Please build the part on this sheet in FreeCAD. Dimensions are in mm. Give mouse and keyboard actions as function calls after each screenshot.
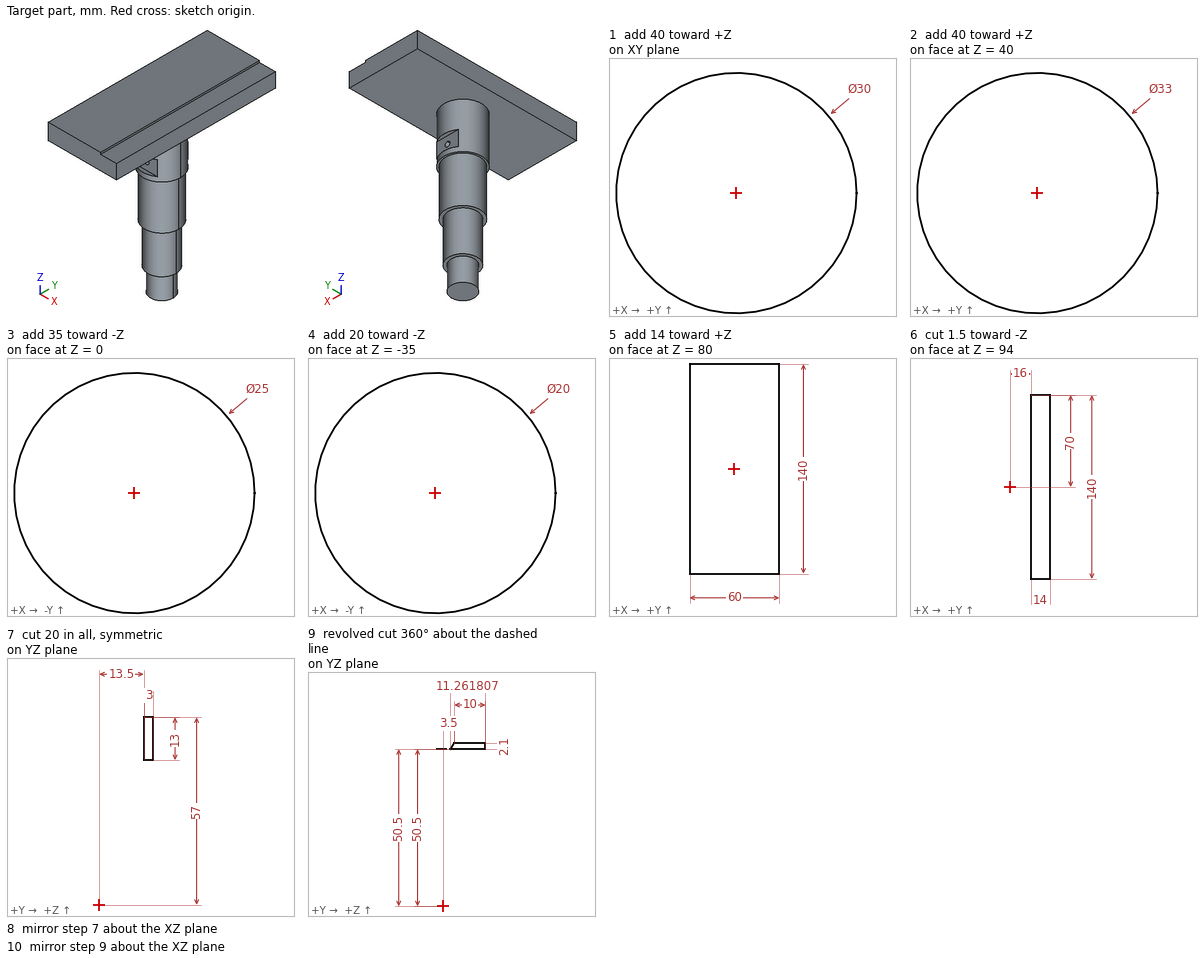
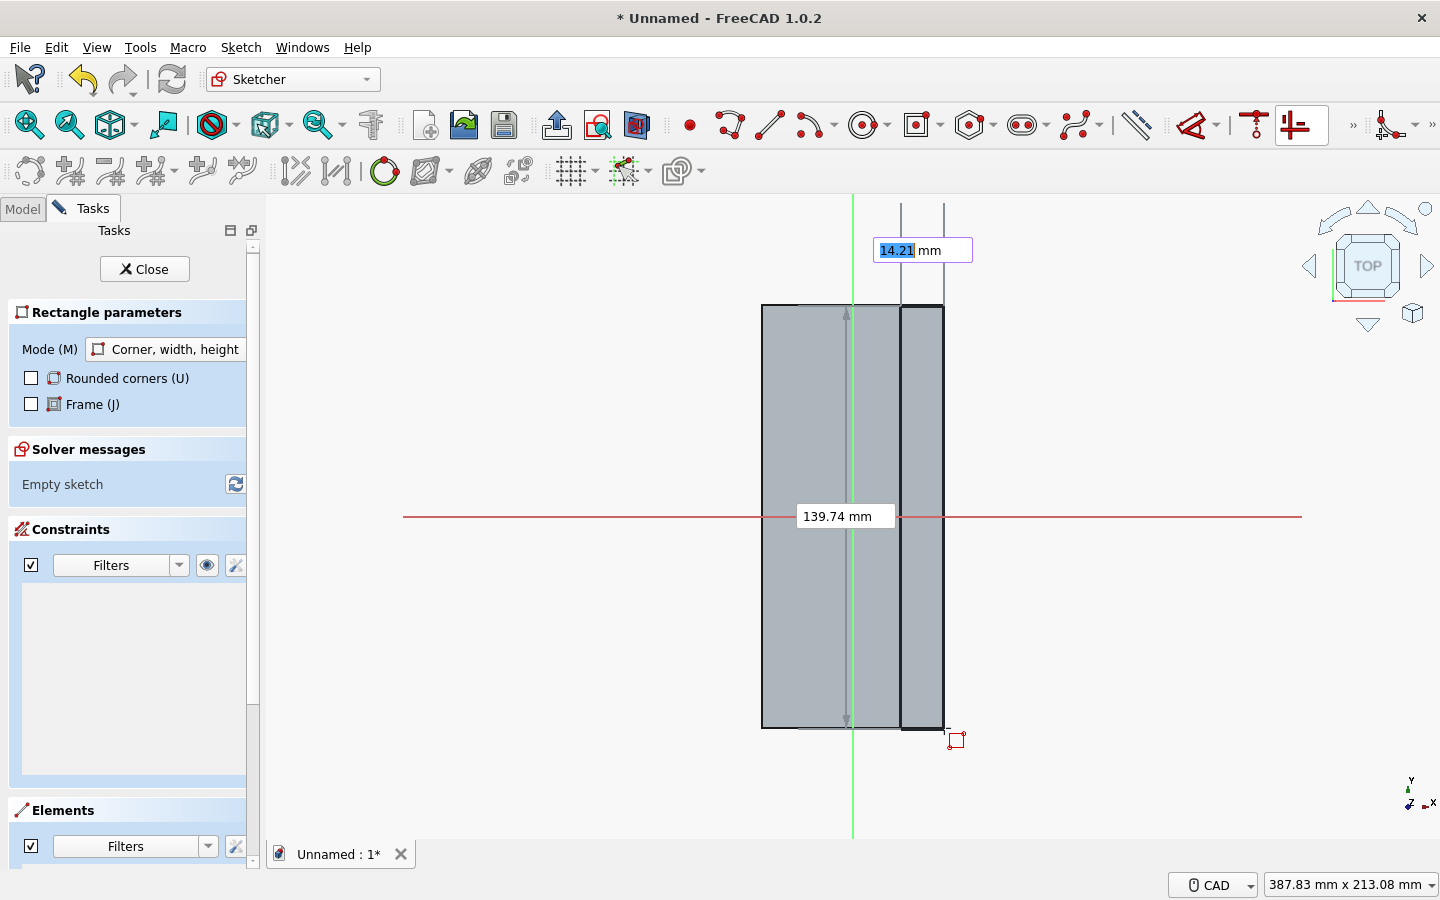
text(14)
key(Tab)
text(140)
key(Return)
key(Escape)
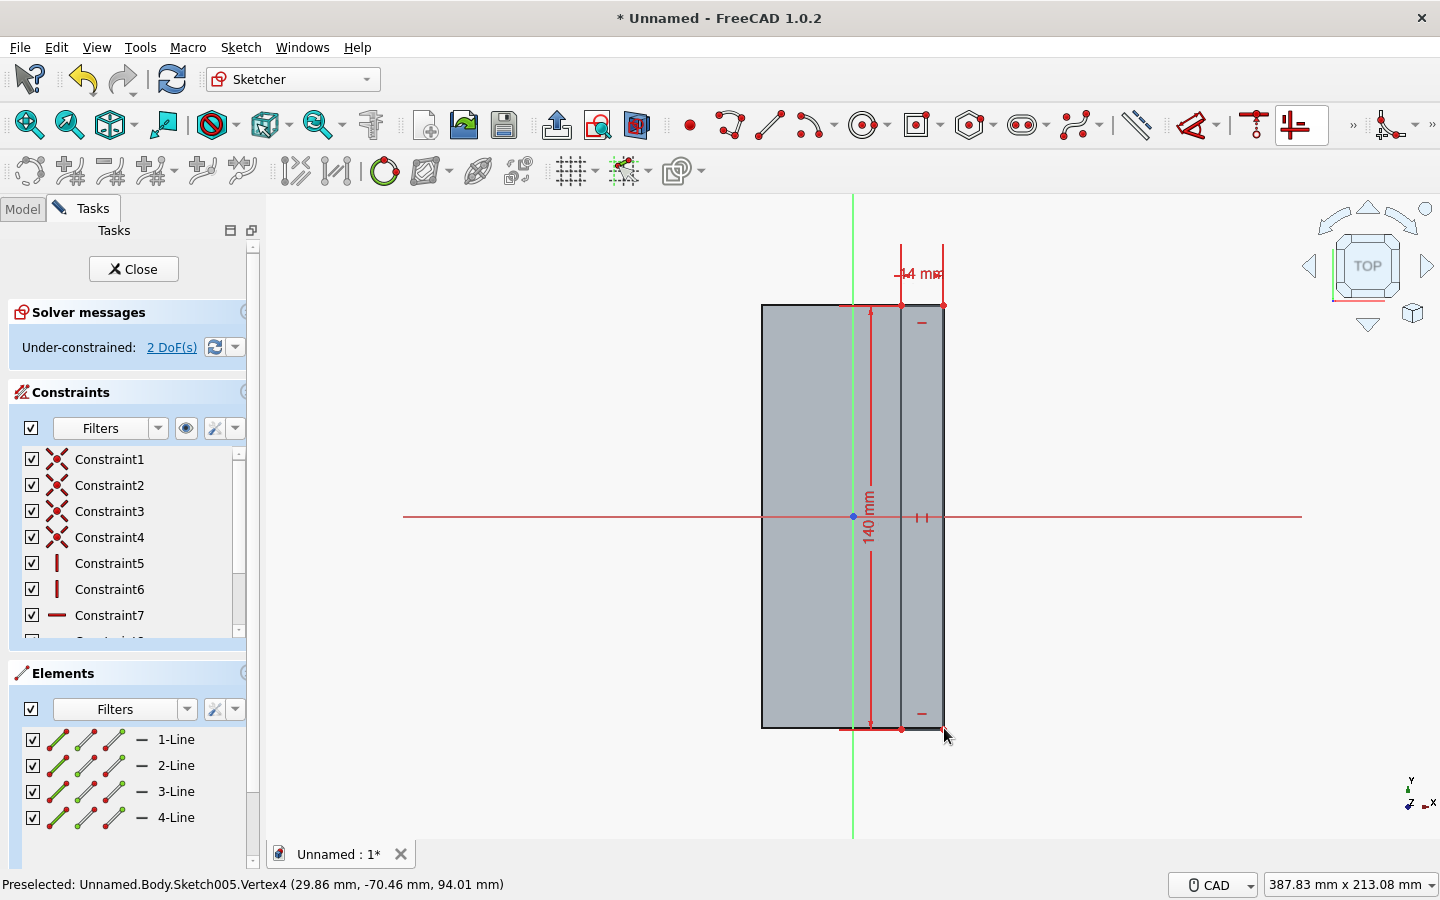
click(1192, 126)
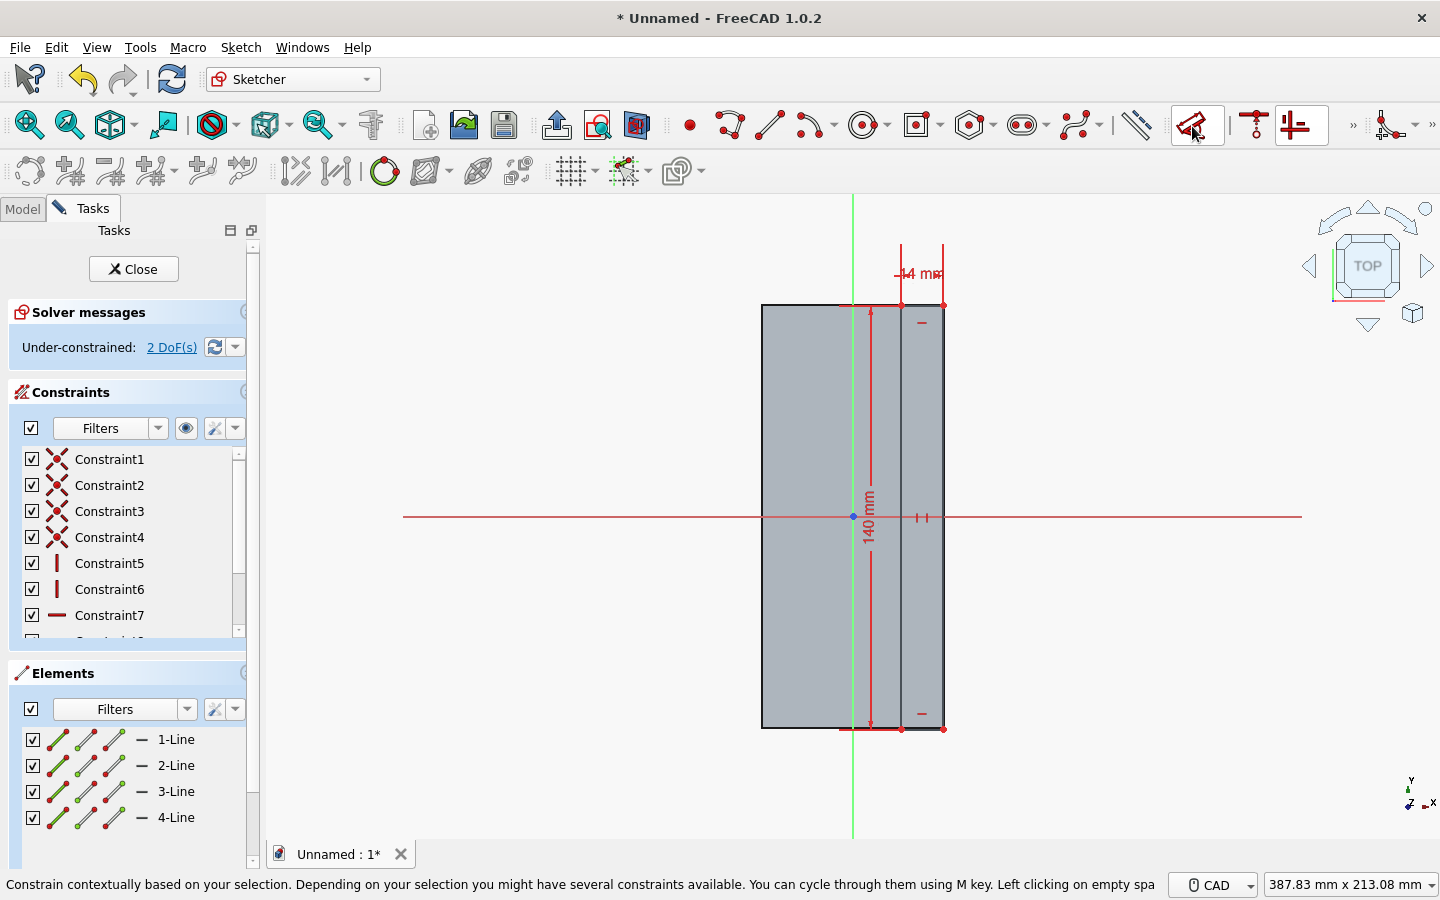
click(901, 306)
click(877, 272)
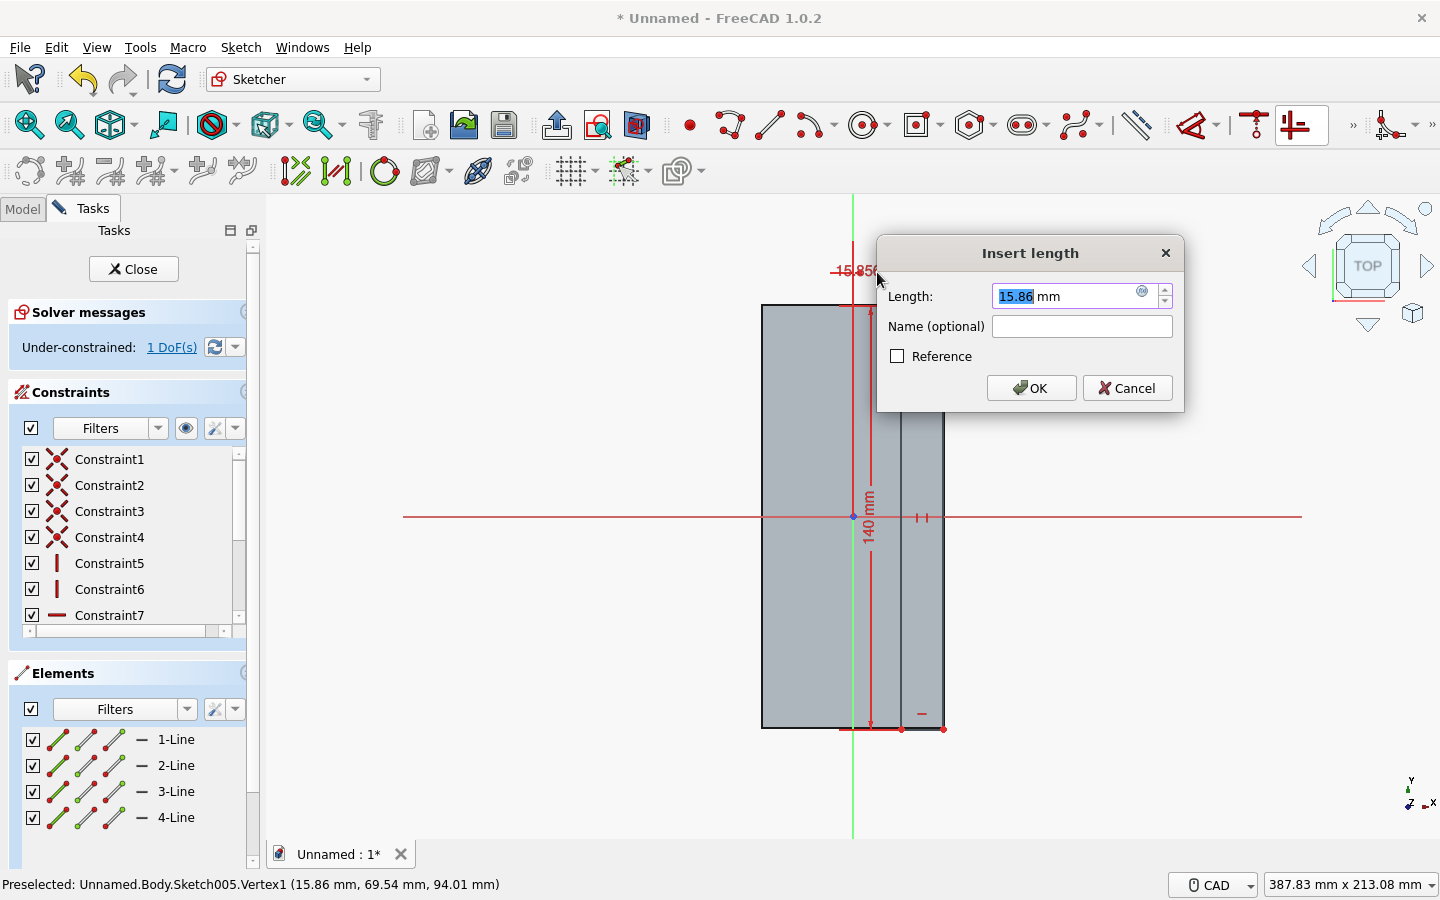
text(16)
key(Return)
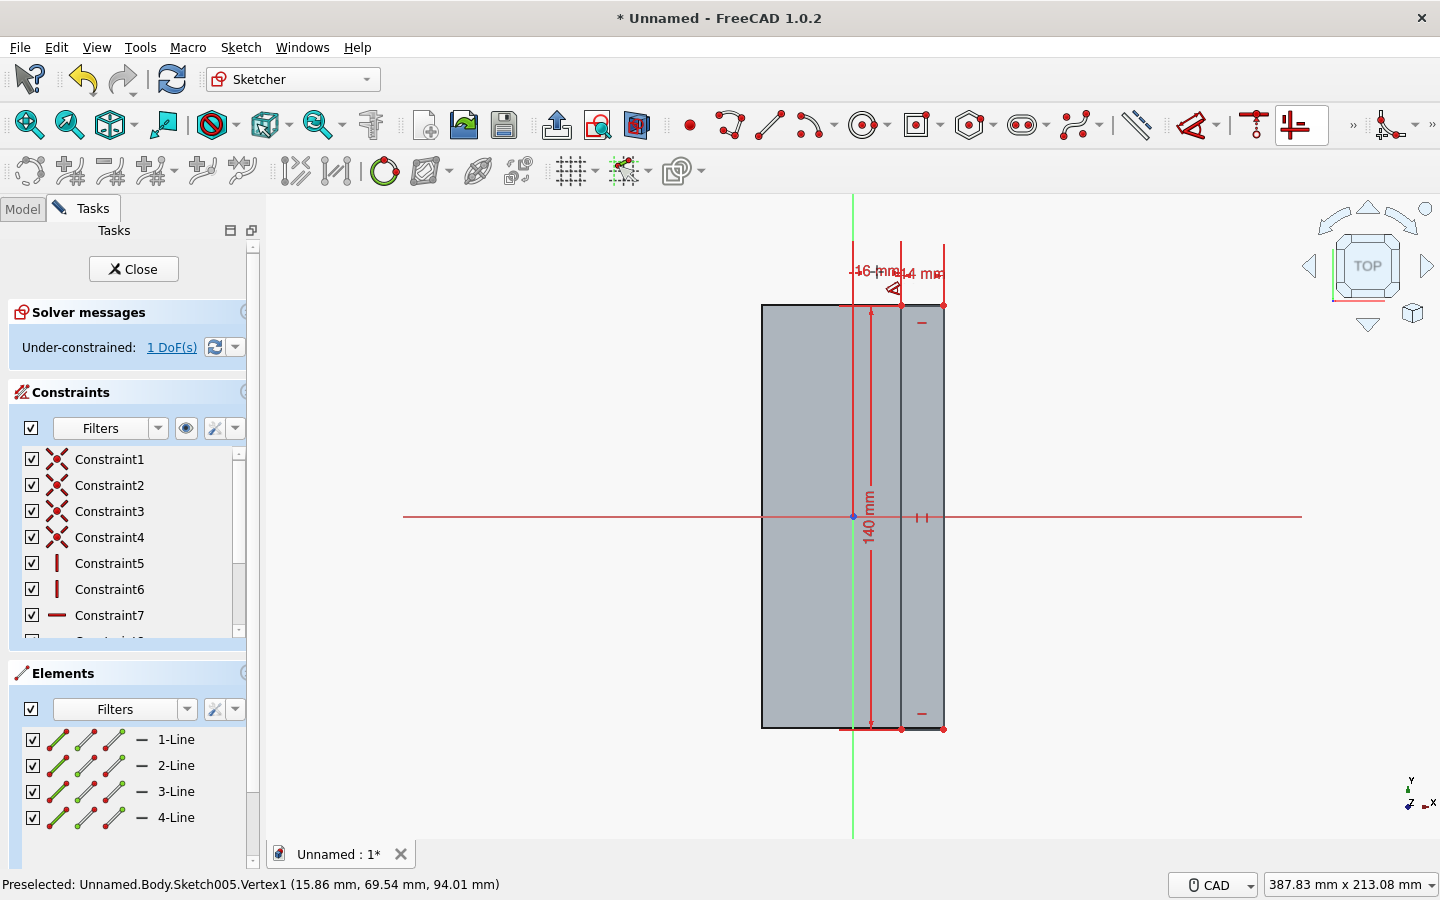
click(901, 306)
click(819, 411)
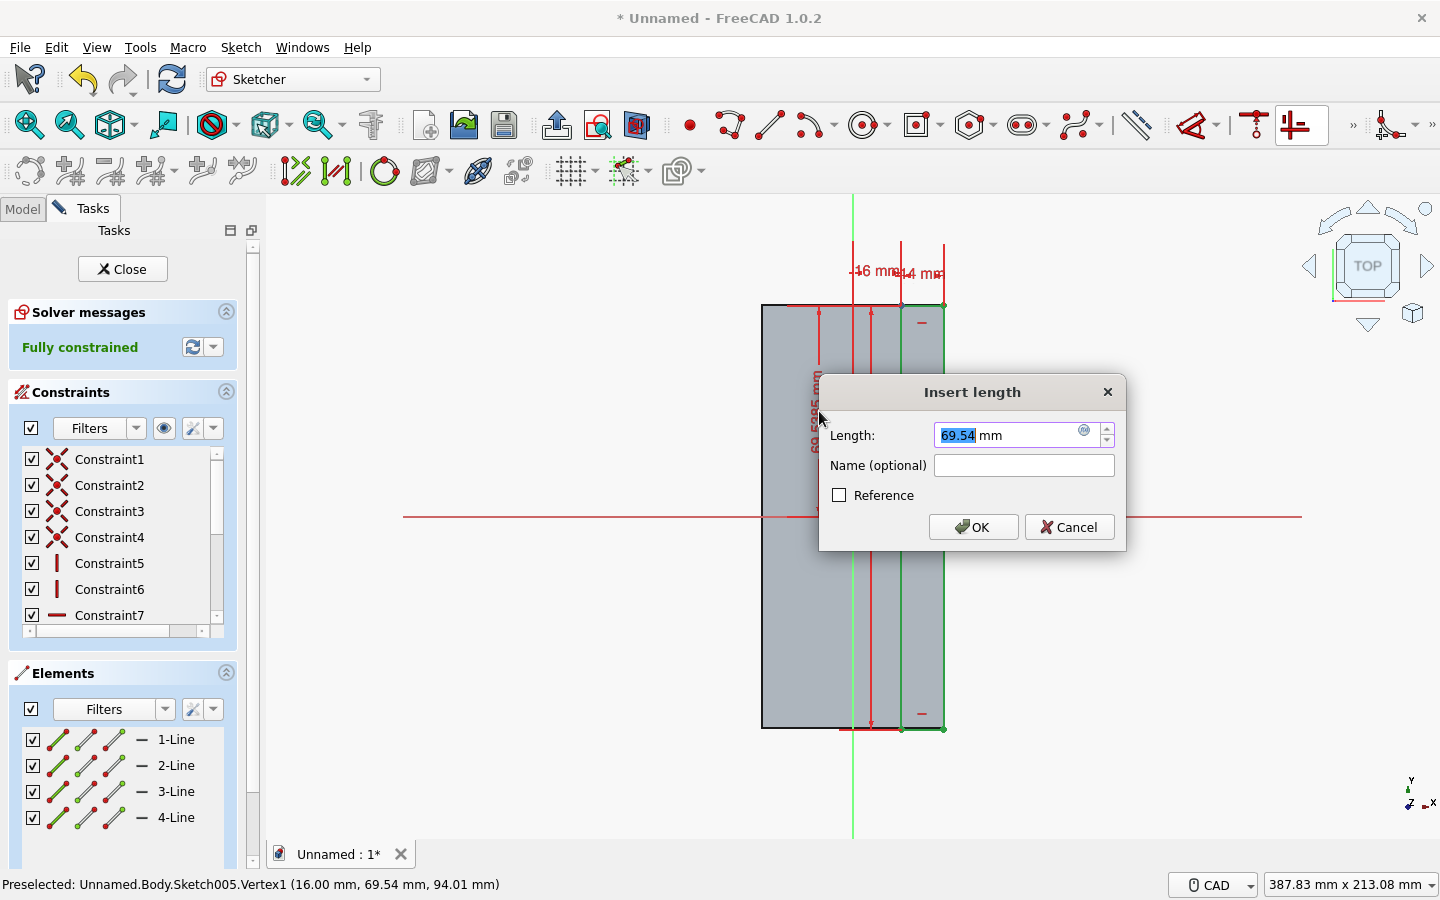
text(70)
key(Return)
key(Escape)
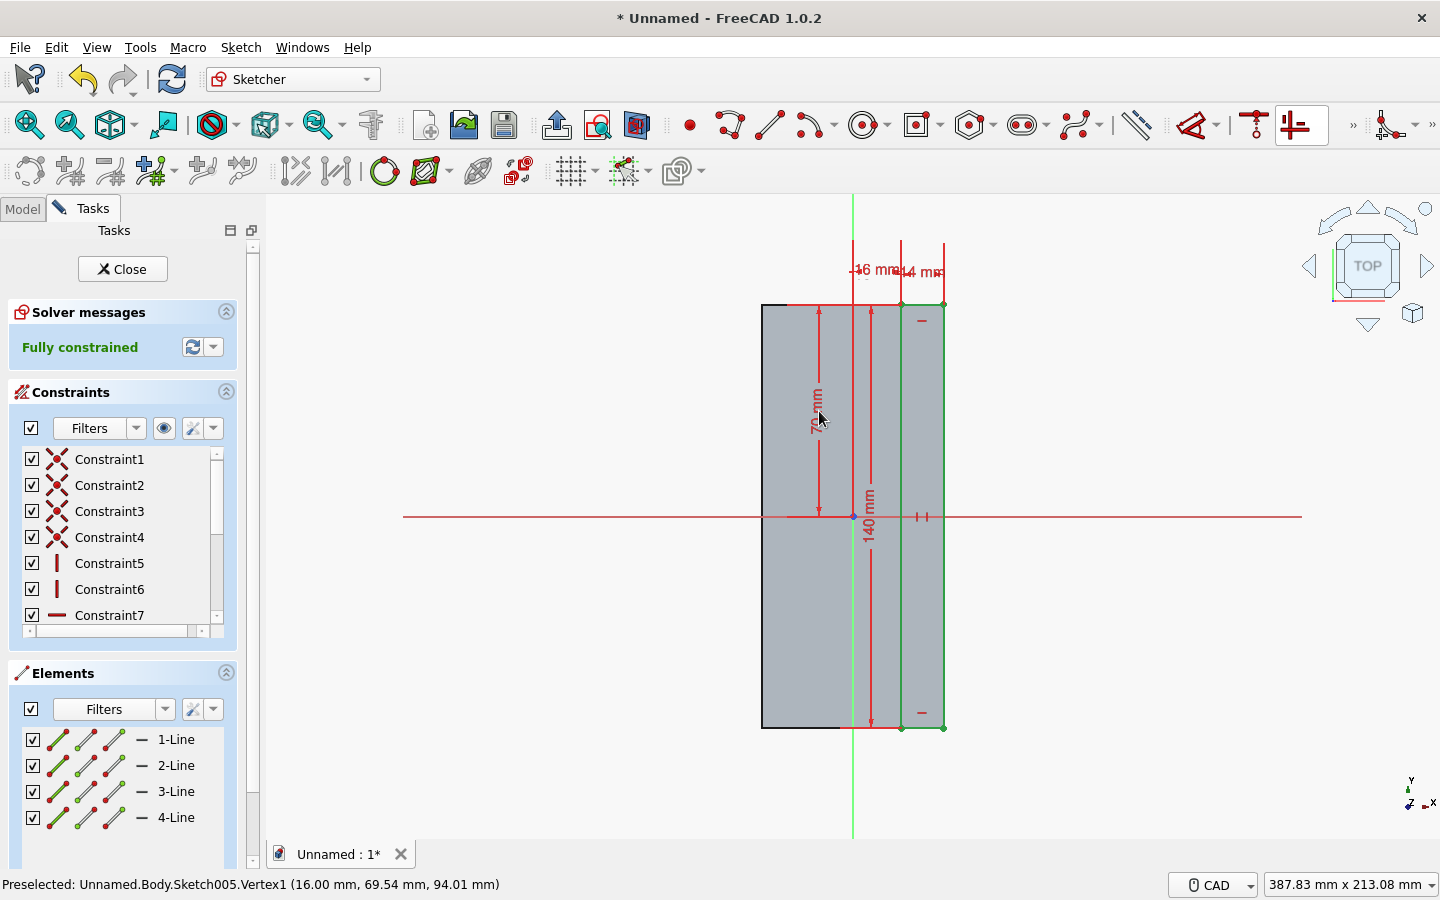
click(123, 269)